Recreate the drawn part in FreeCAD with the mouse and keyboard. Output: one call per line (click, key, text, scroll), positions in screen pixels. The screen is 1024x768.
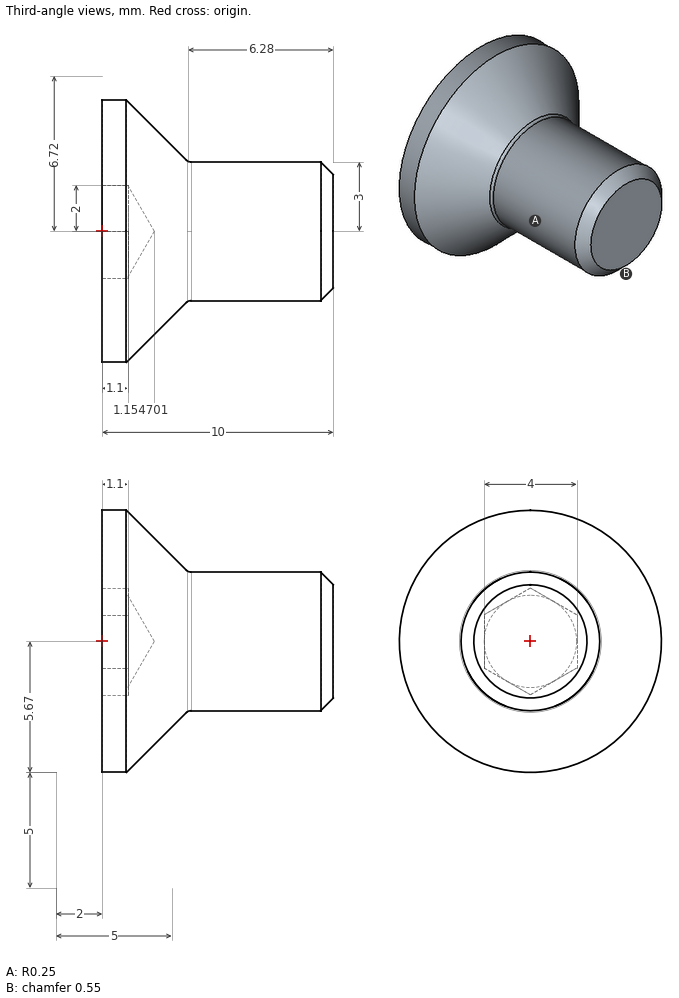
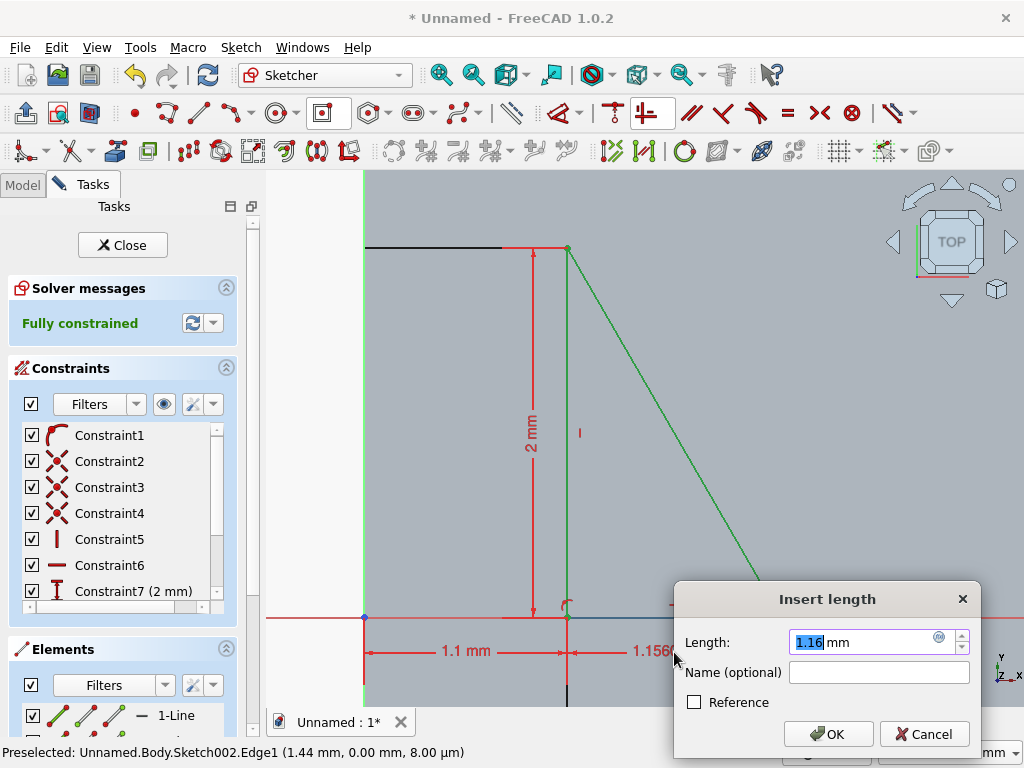
text(1.154701)
key(Return)
key(Escape)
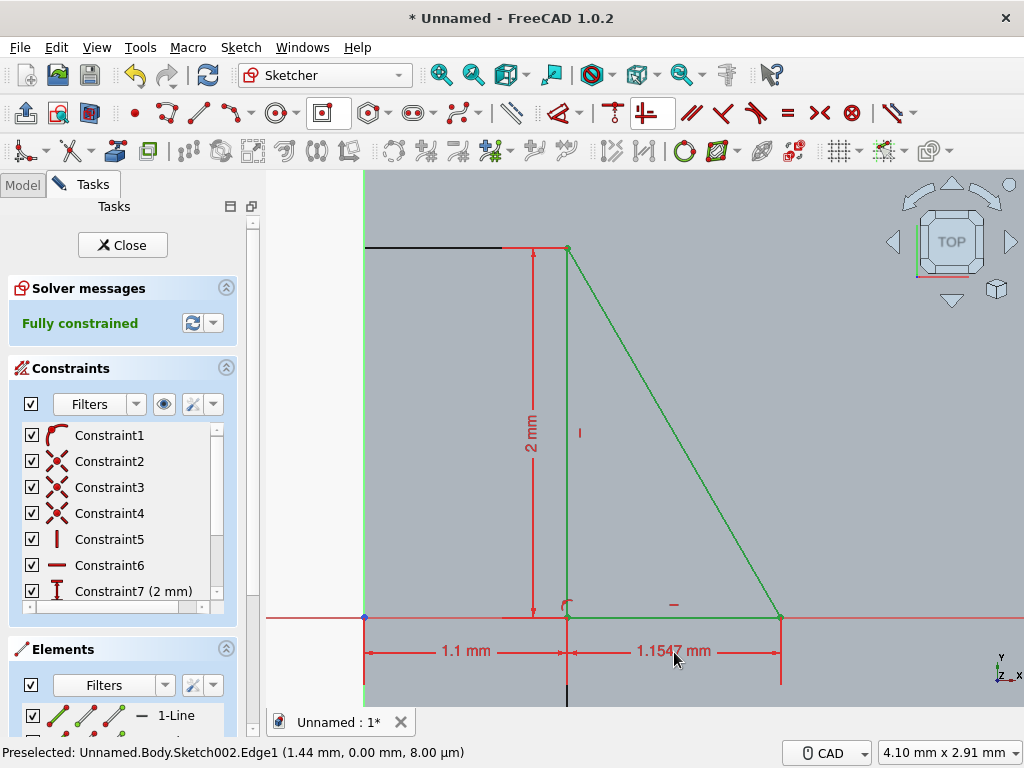
click(123, 245)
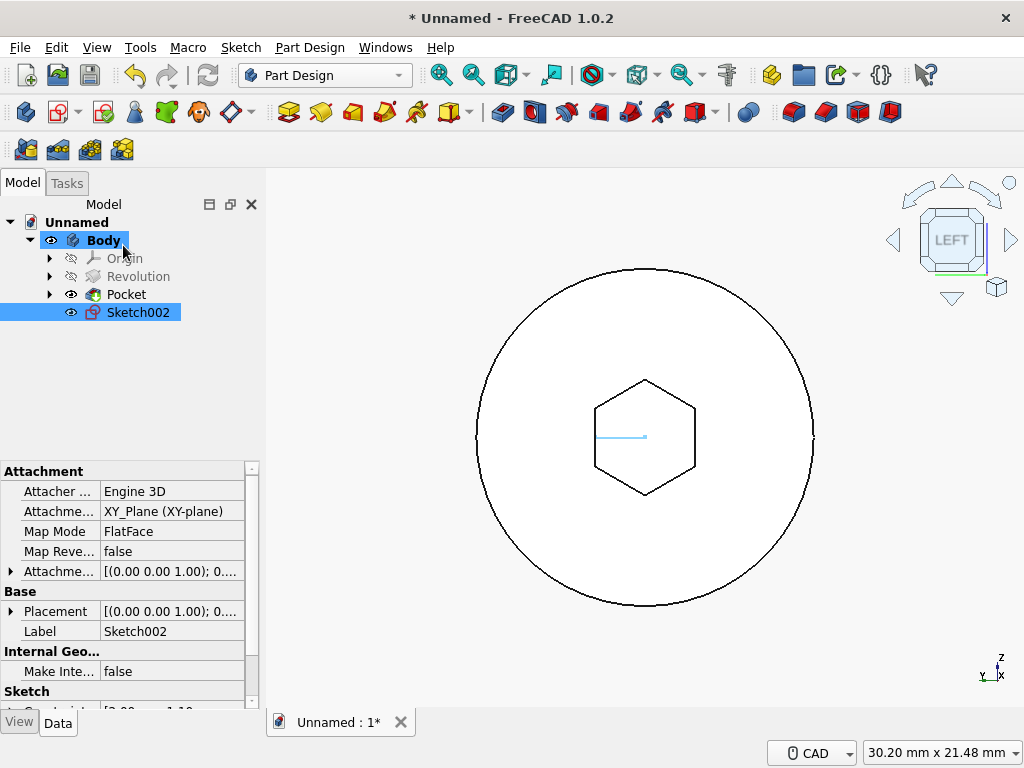
click(568, 112)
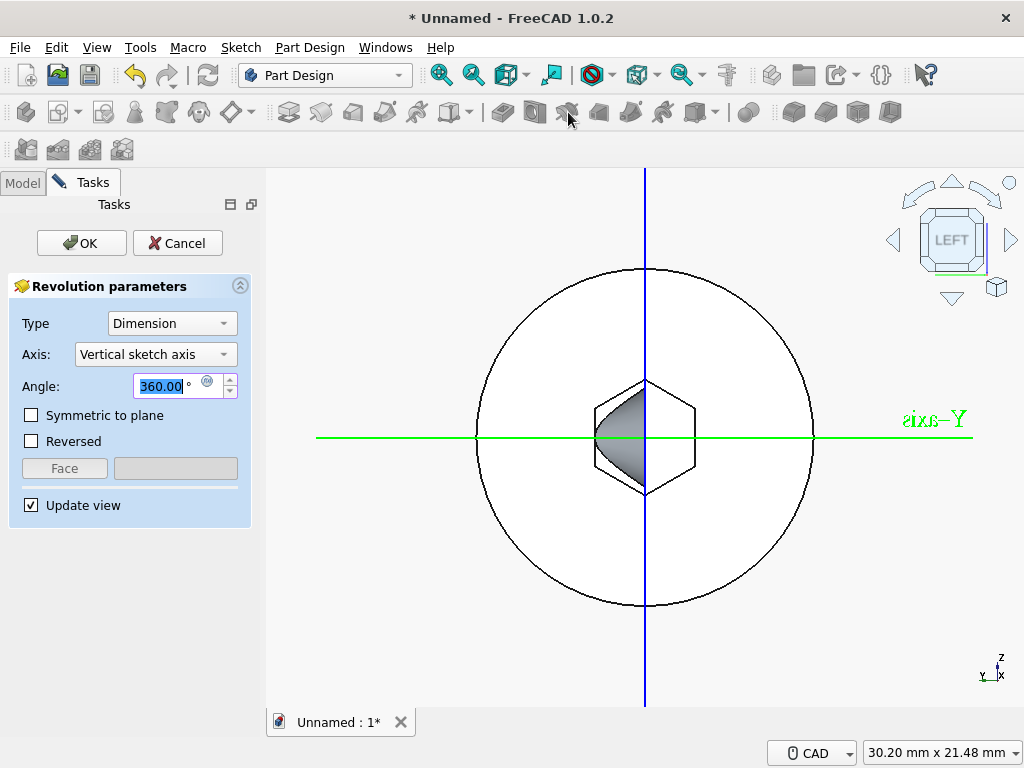
click(156, 354)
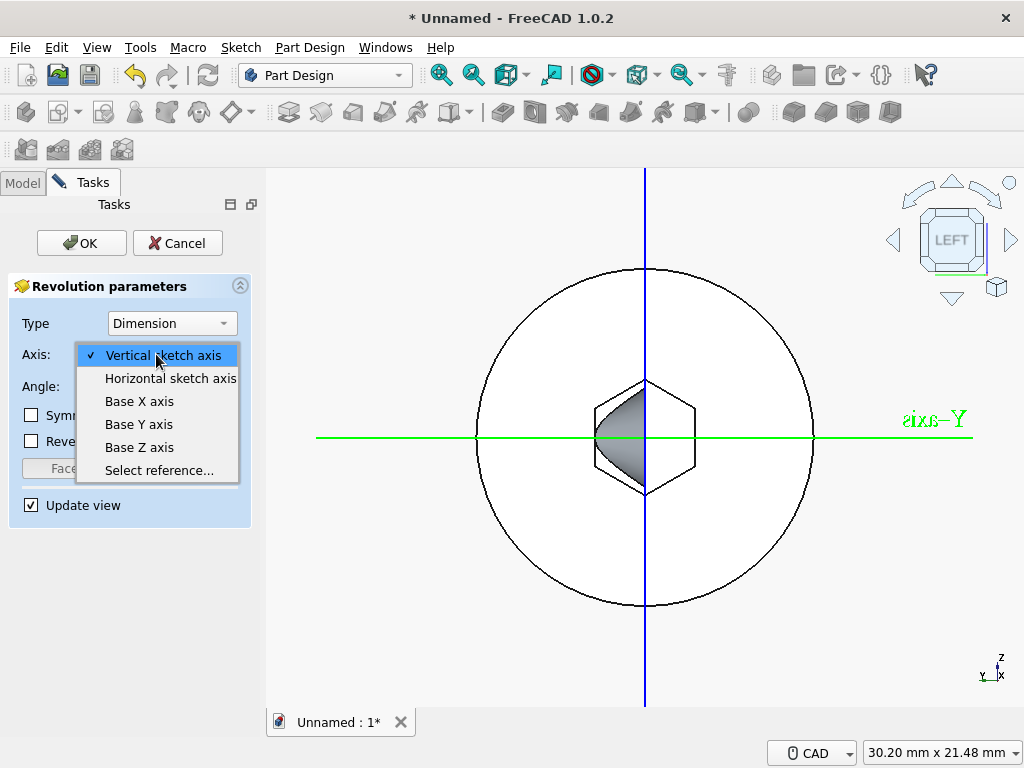
click(156, 378)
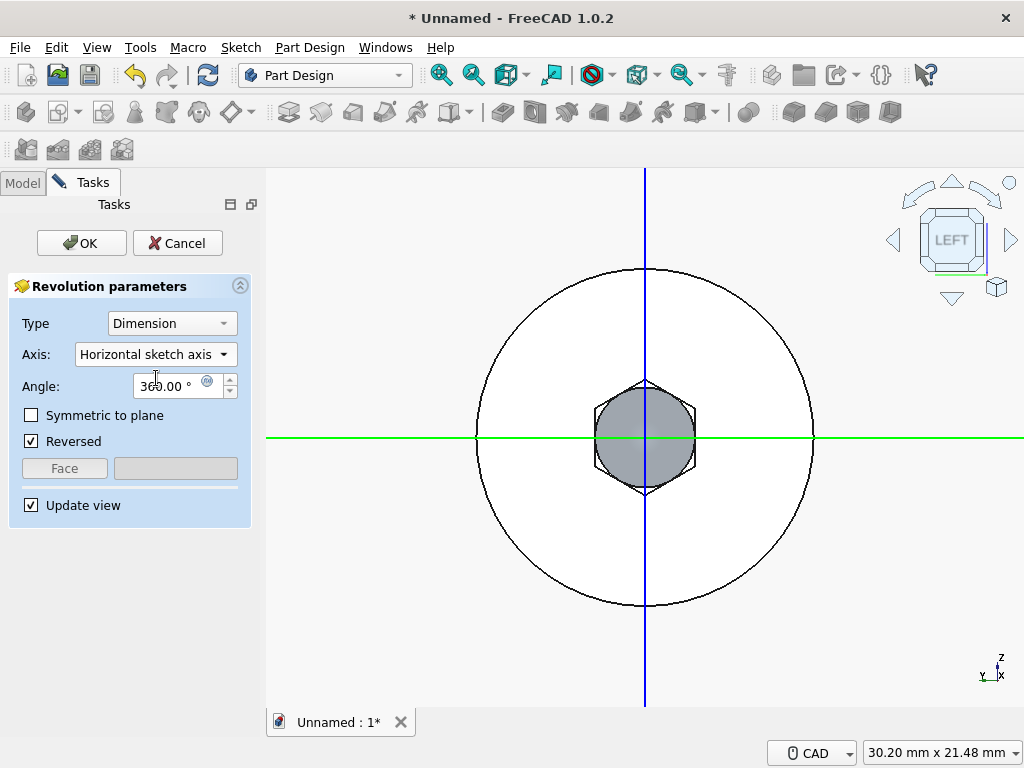
click(82, 243)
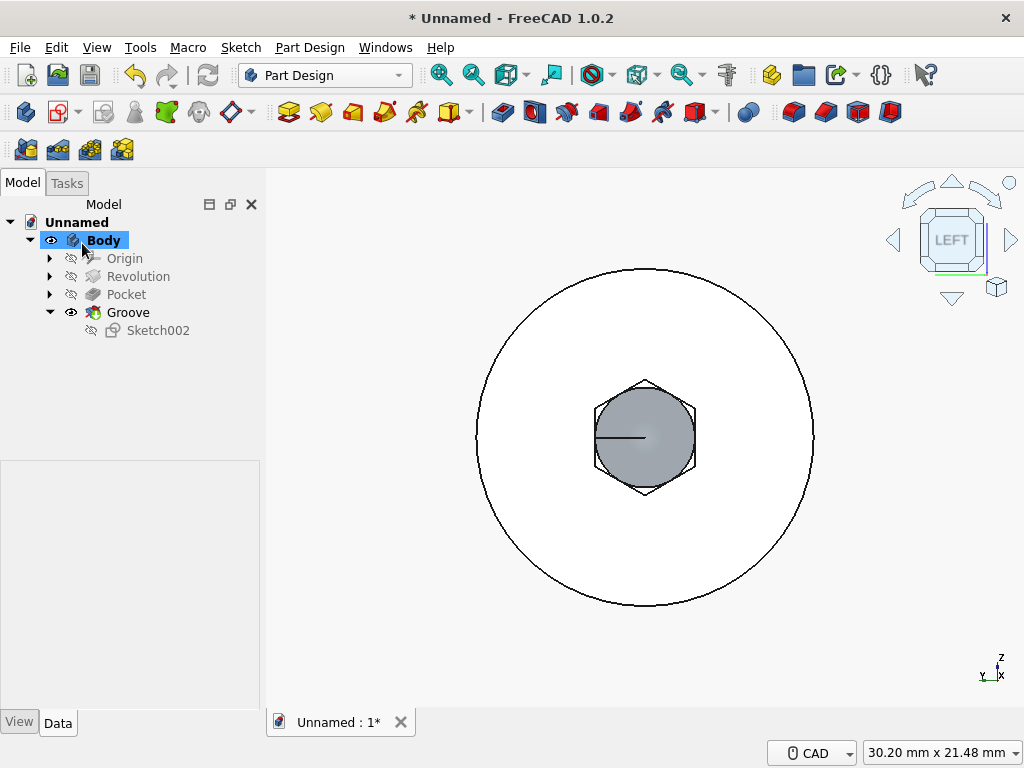
key(0)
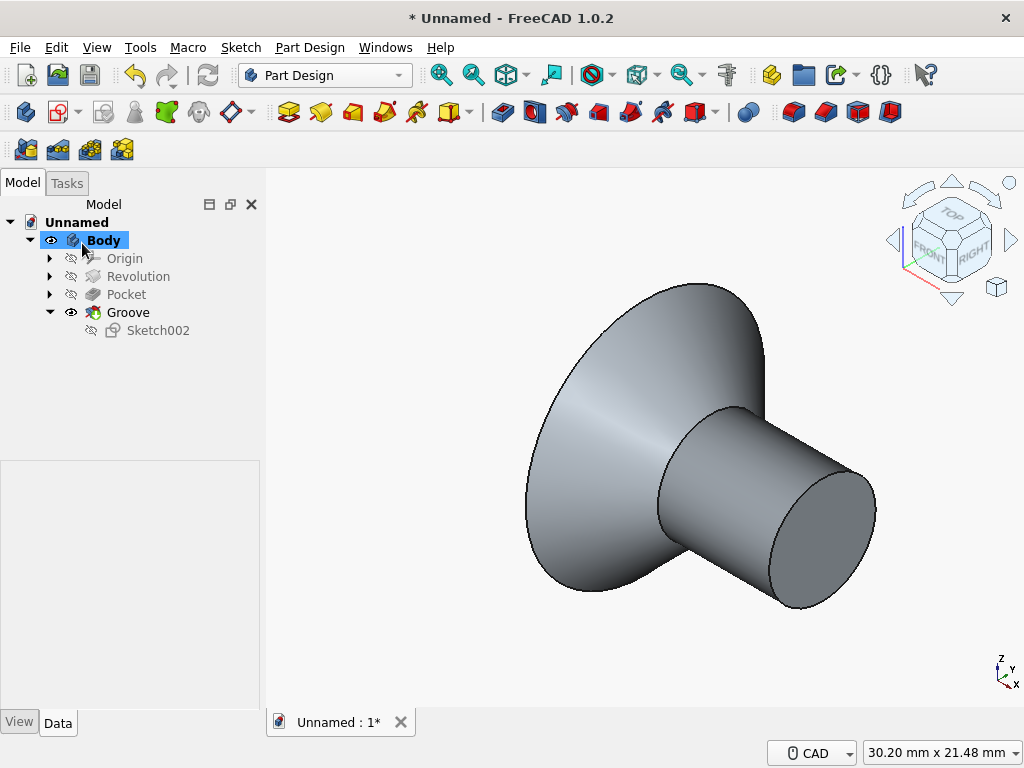
key(v)
key(f)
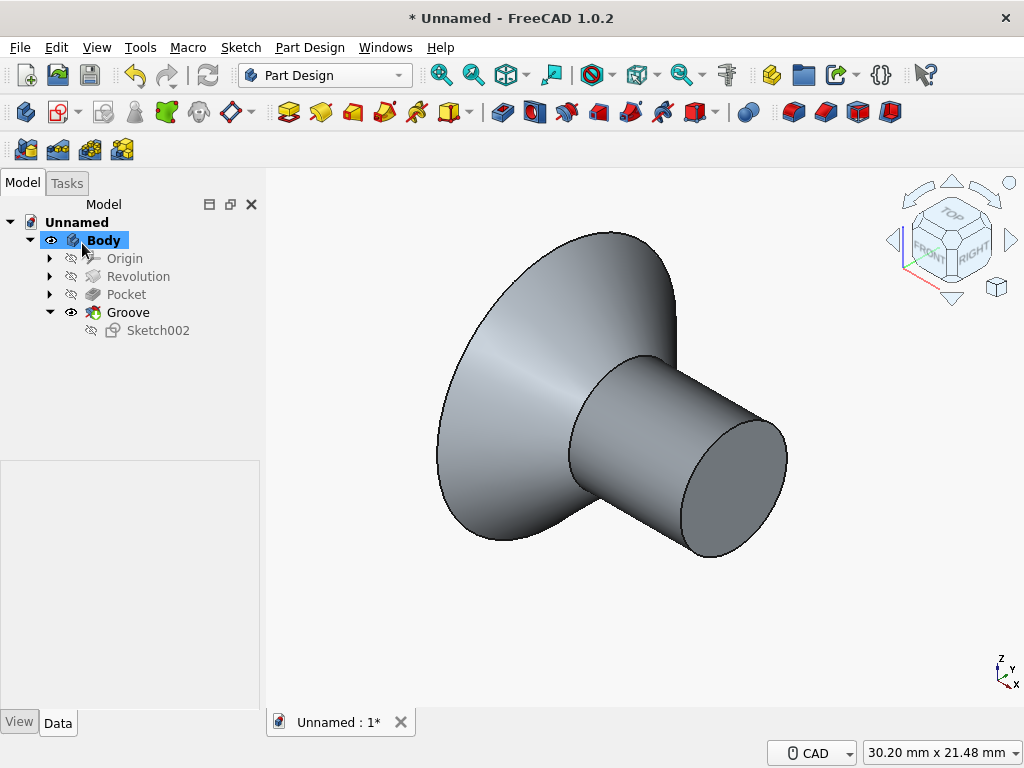
key(2)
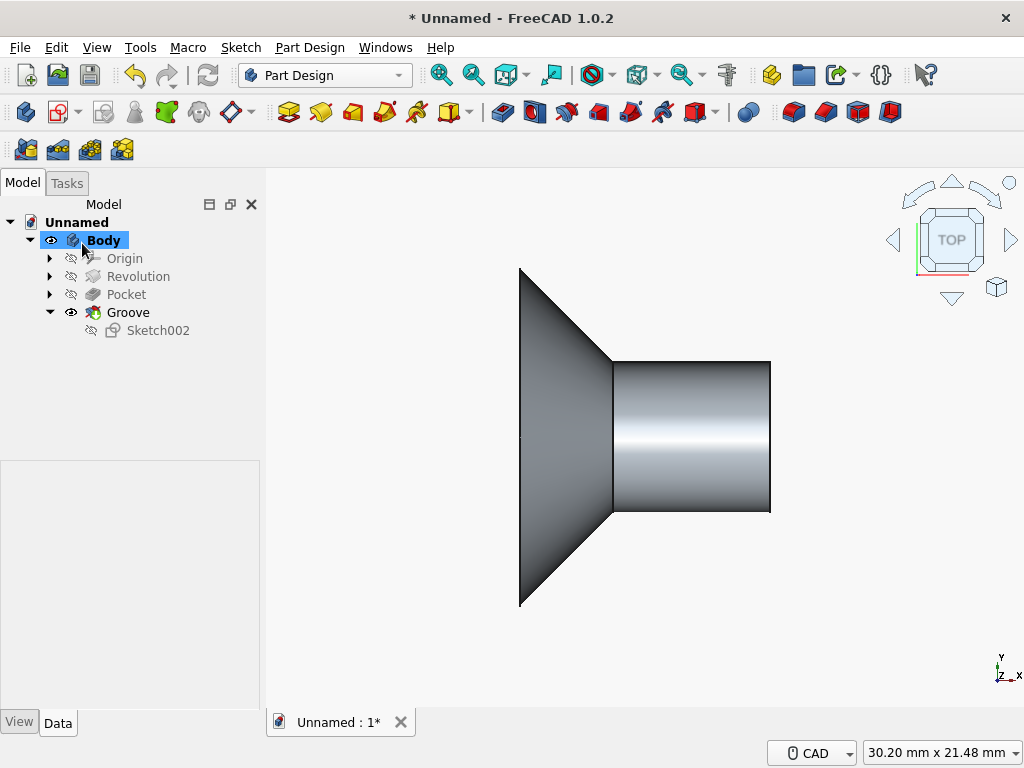
key(1)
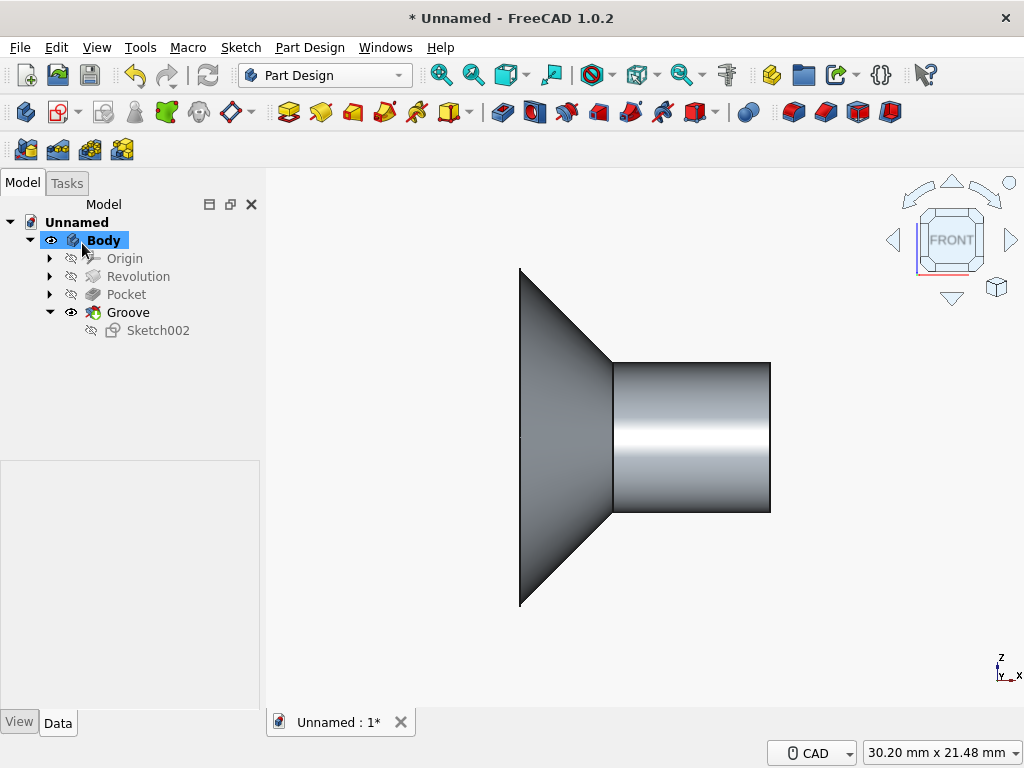
key(3)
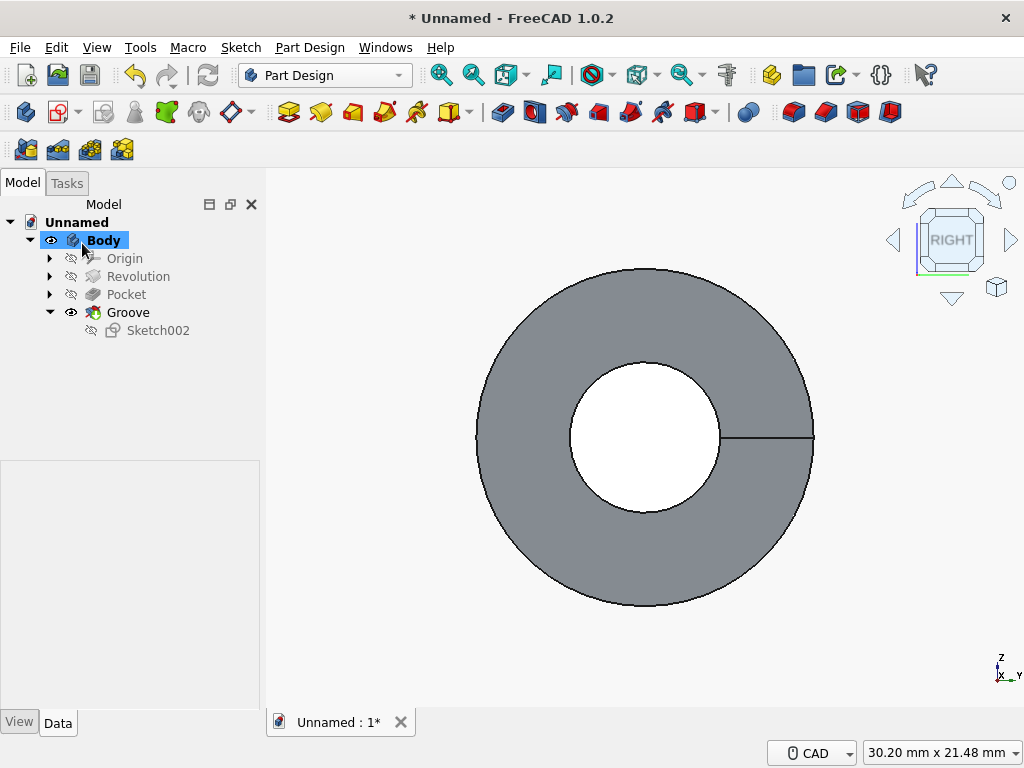
key(5)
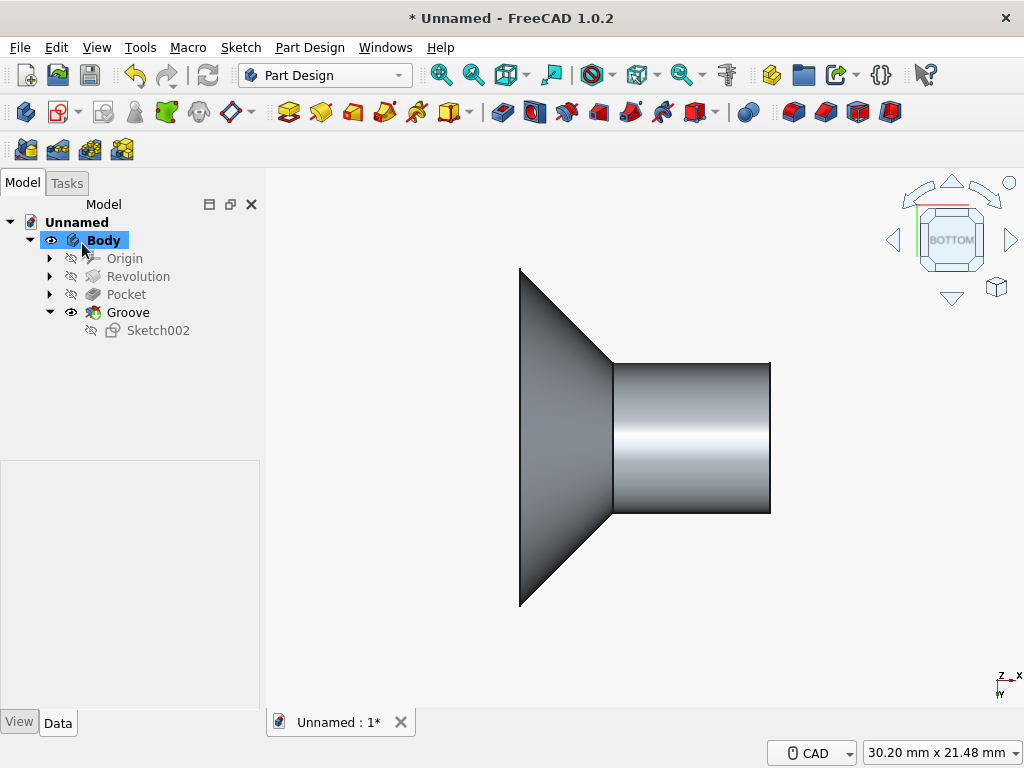
key(4)